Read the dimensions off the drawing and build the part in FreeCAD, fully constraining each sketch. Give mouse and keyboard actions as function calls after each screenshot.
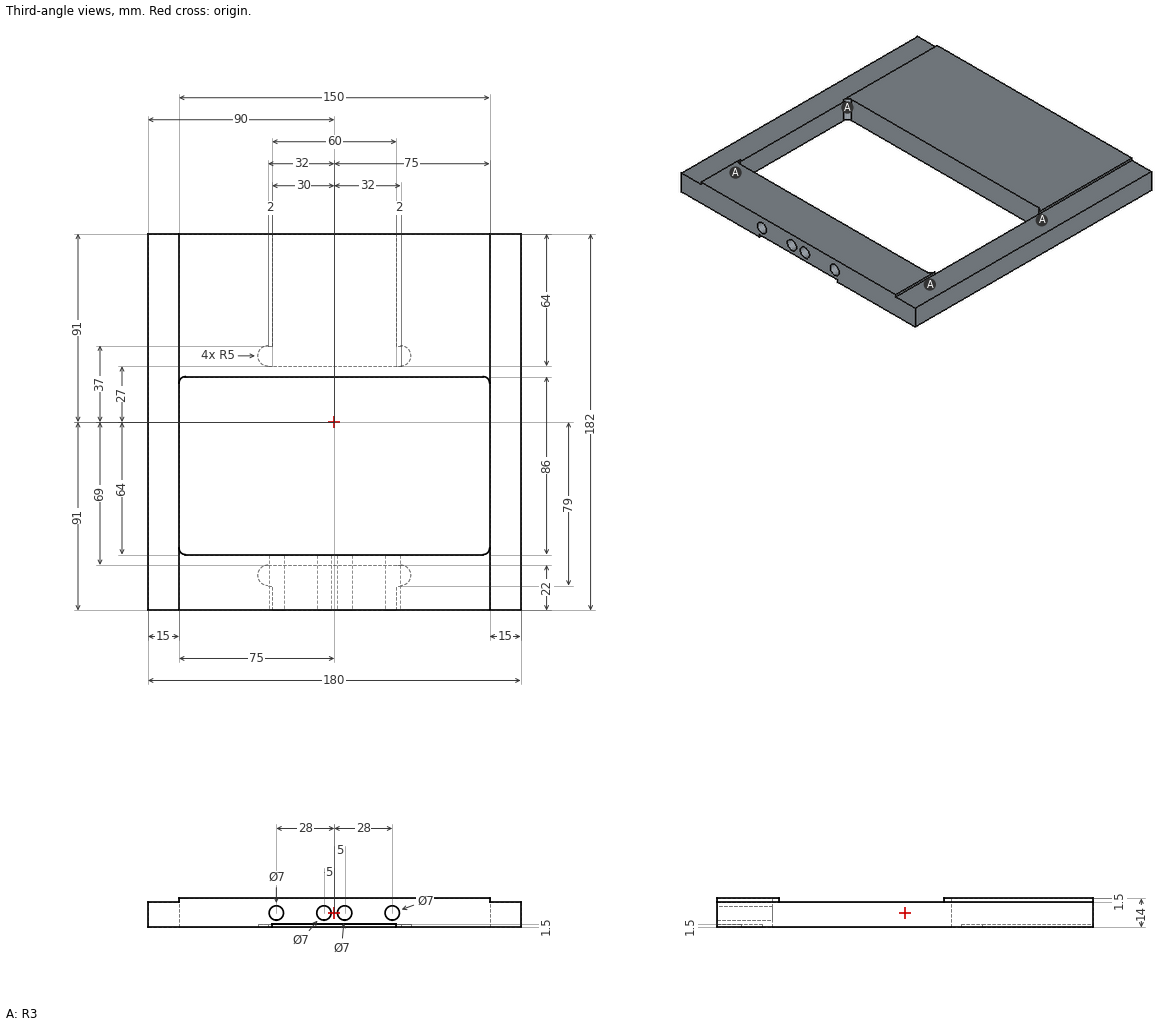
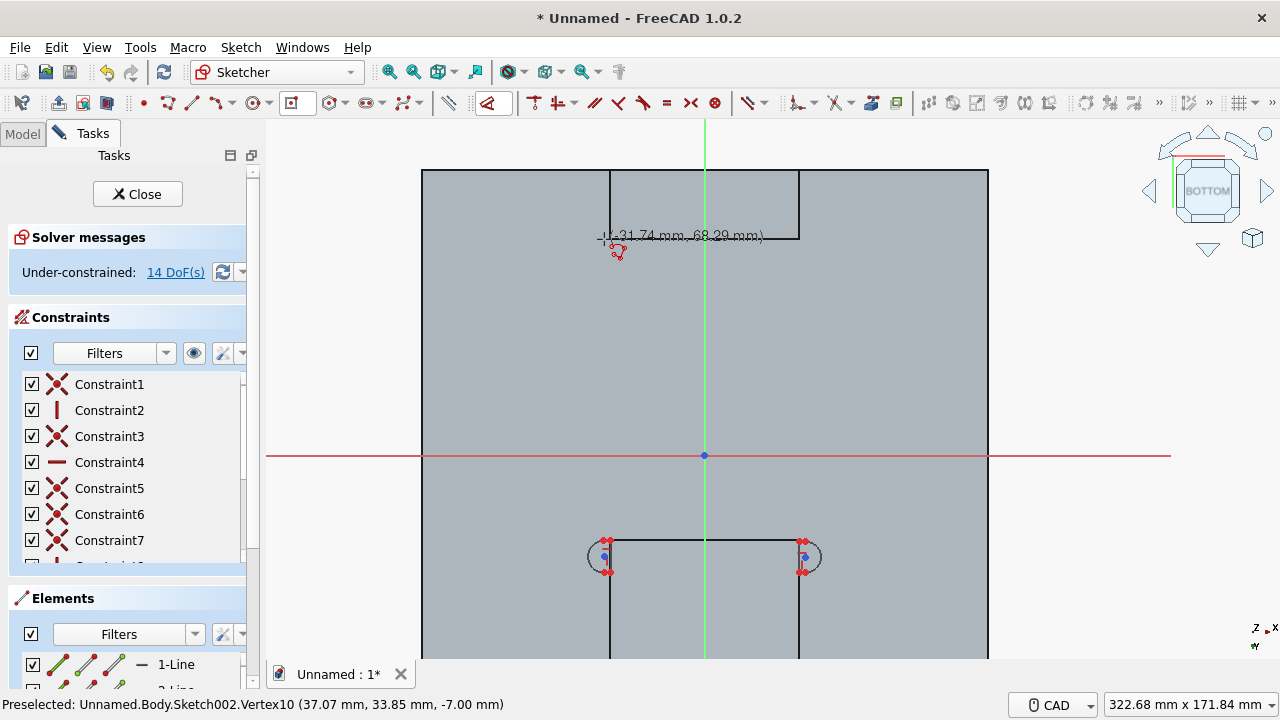
scroll(610, 239, up, 5)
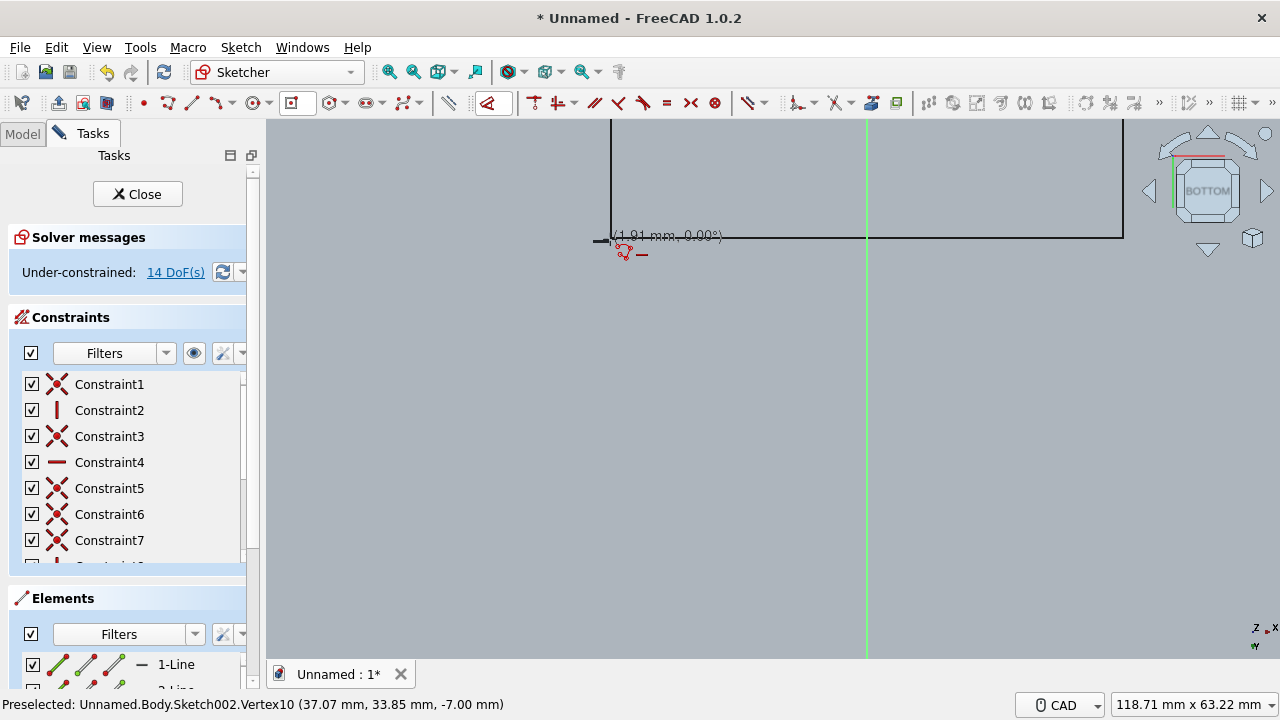
click(611, 239)
click(611, 153)
click(594, 153)
right_click(594, 153)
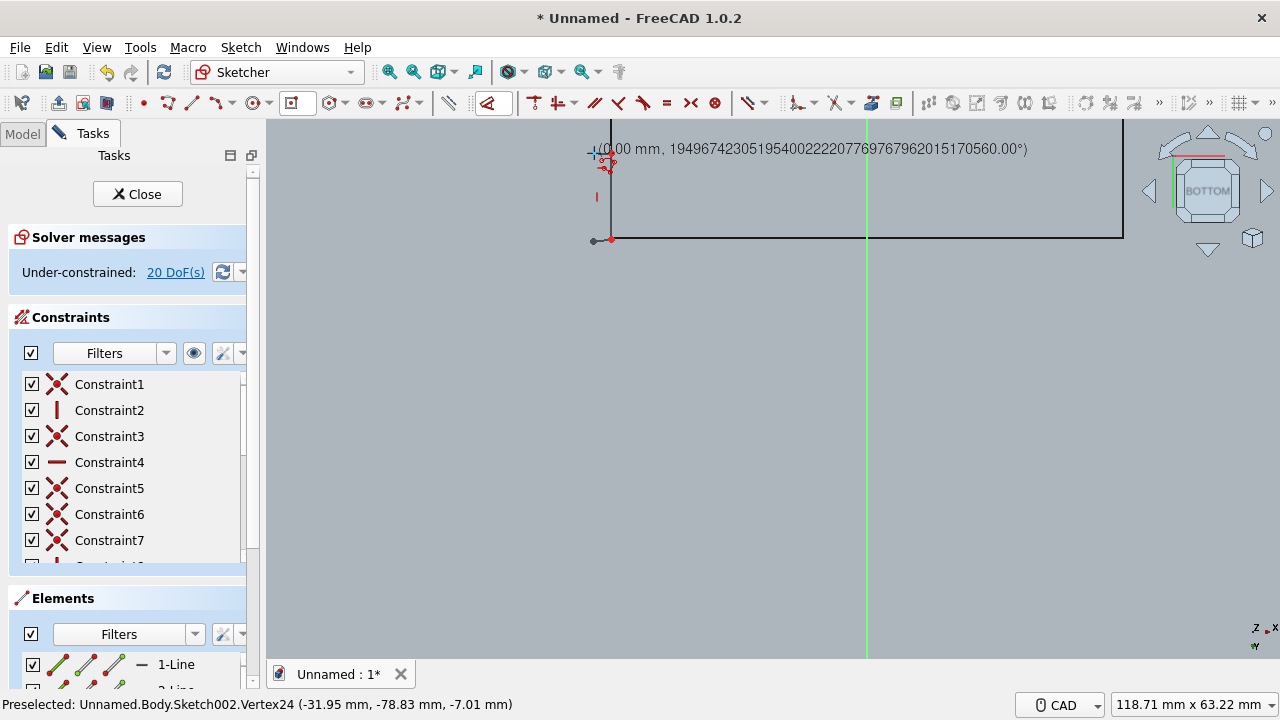
key(g)
key(3)
key(a)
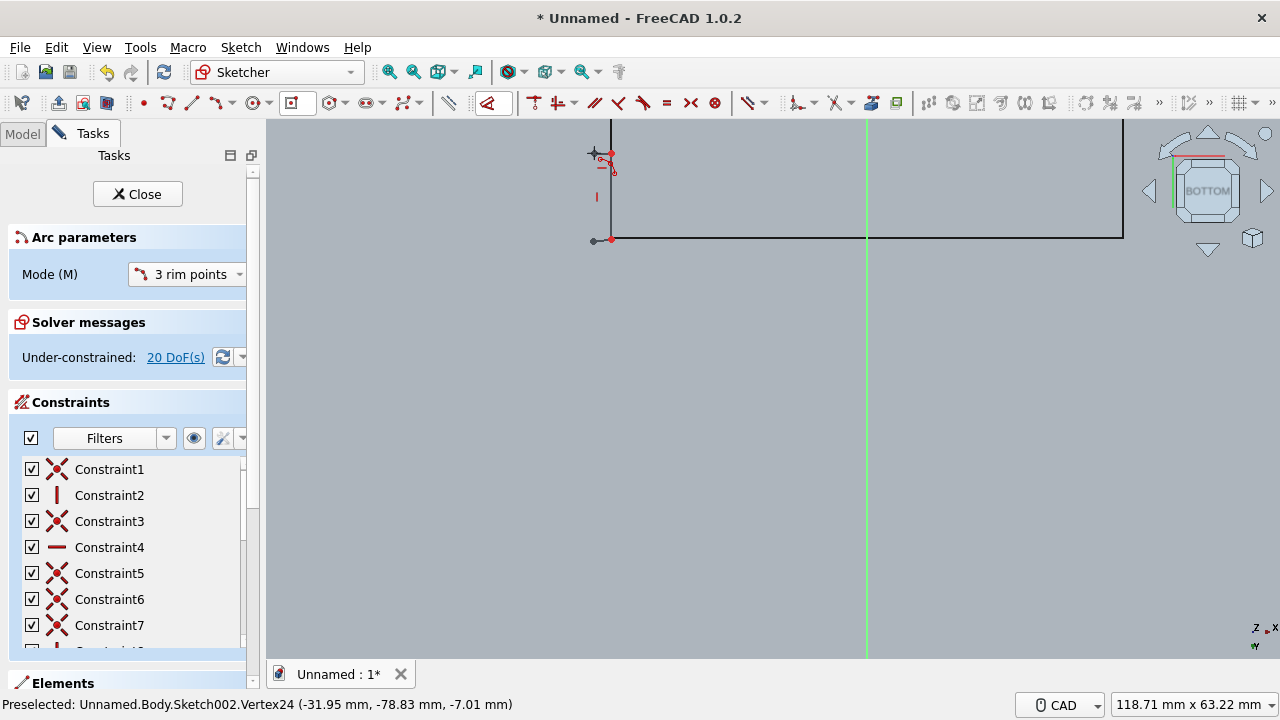
scroll(594, 153, up, 4)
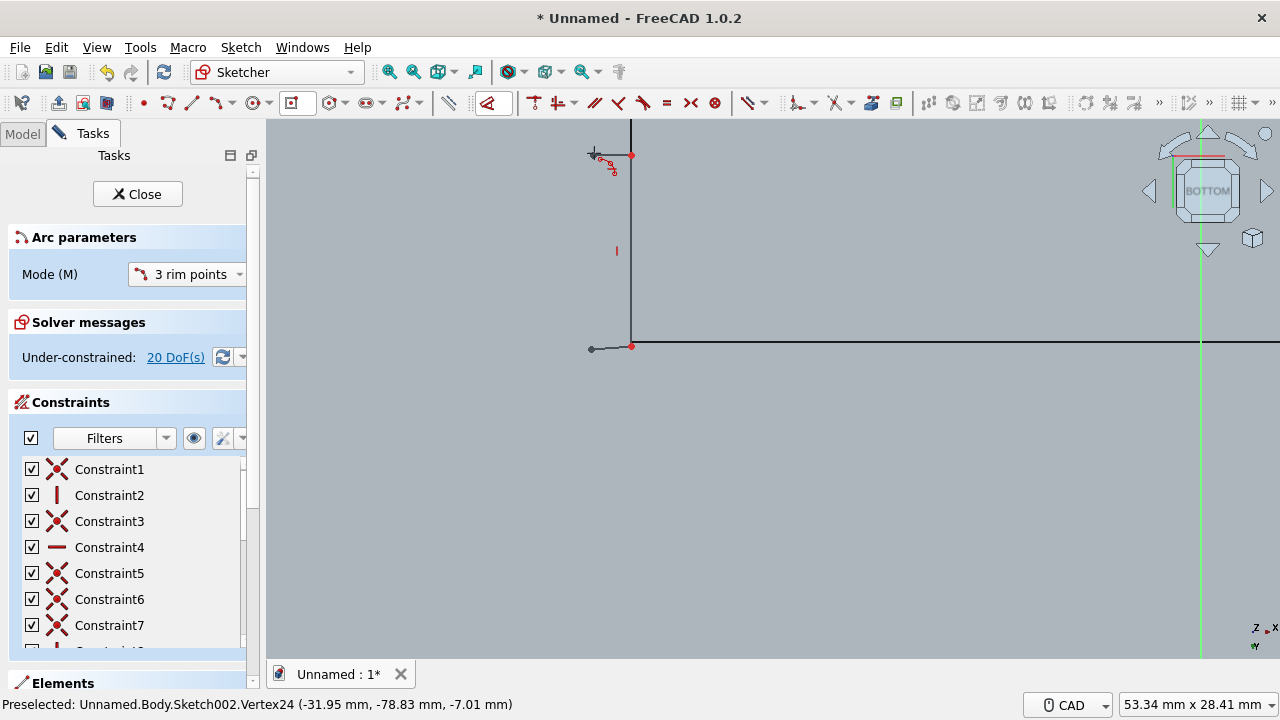
click(594, 155)
click(592, 350)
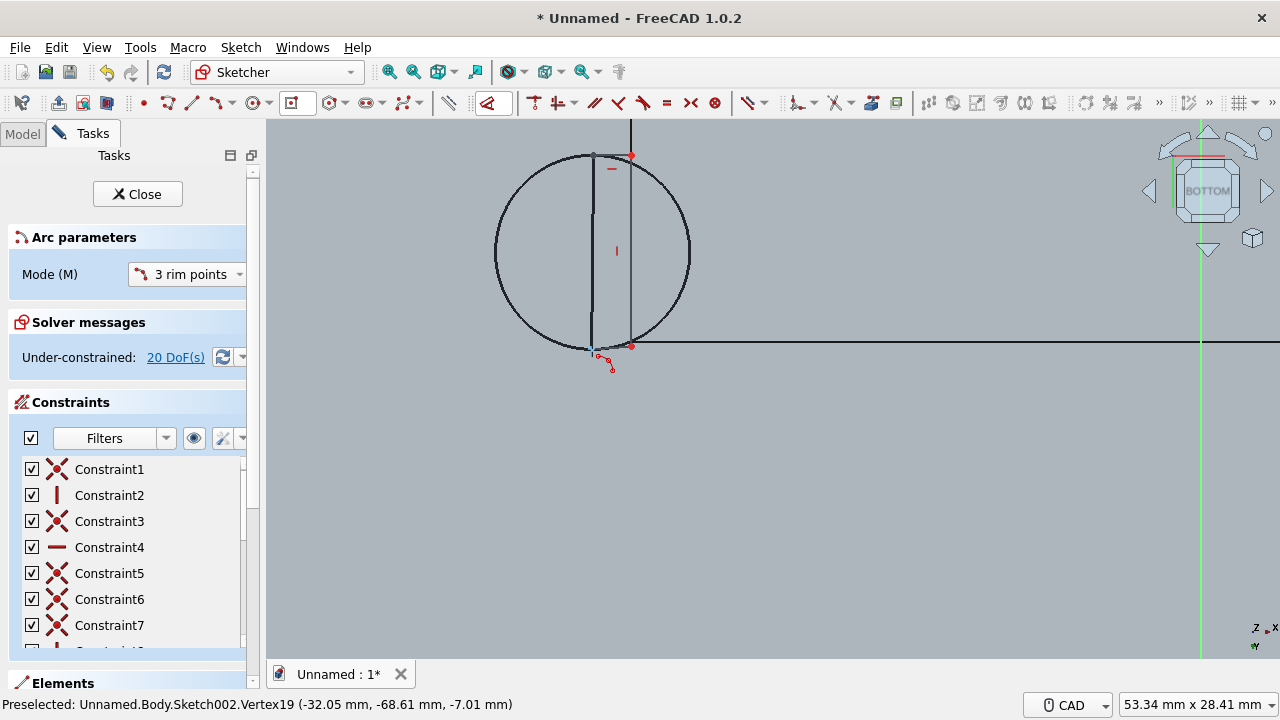
scroll(606, 218, down, 9)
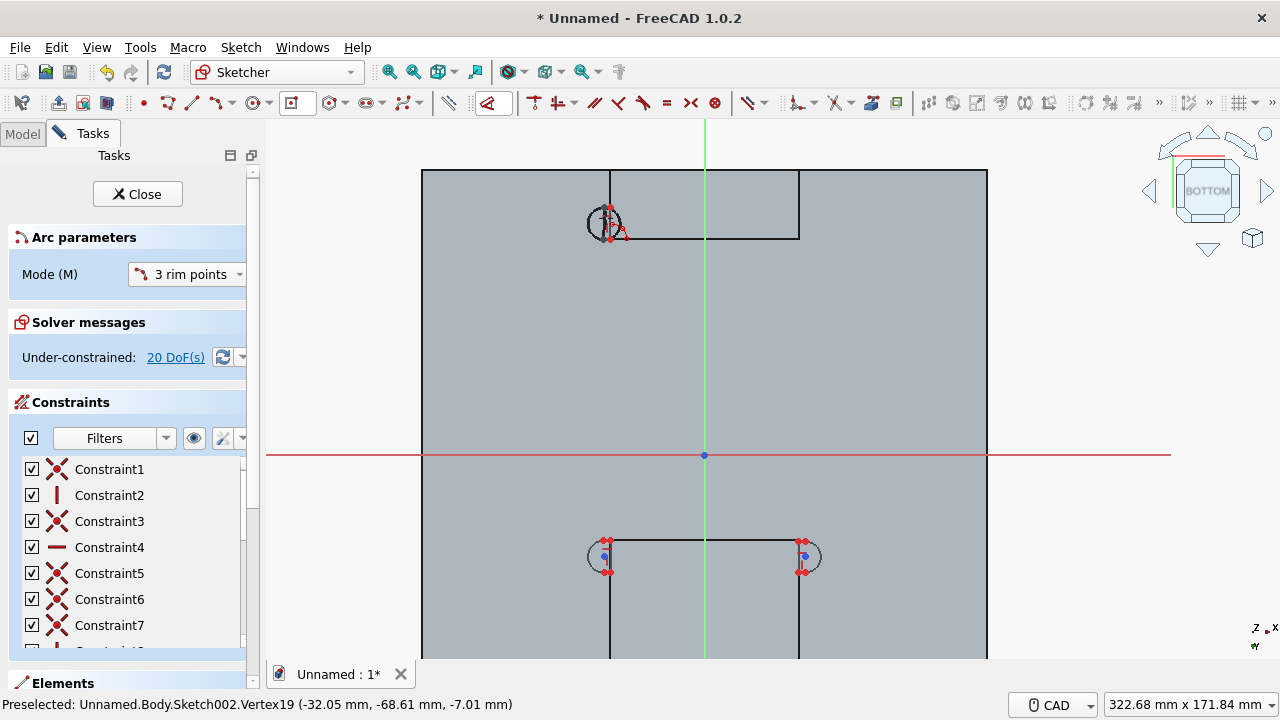
click(588, 223)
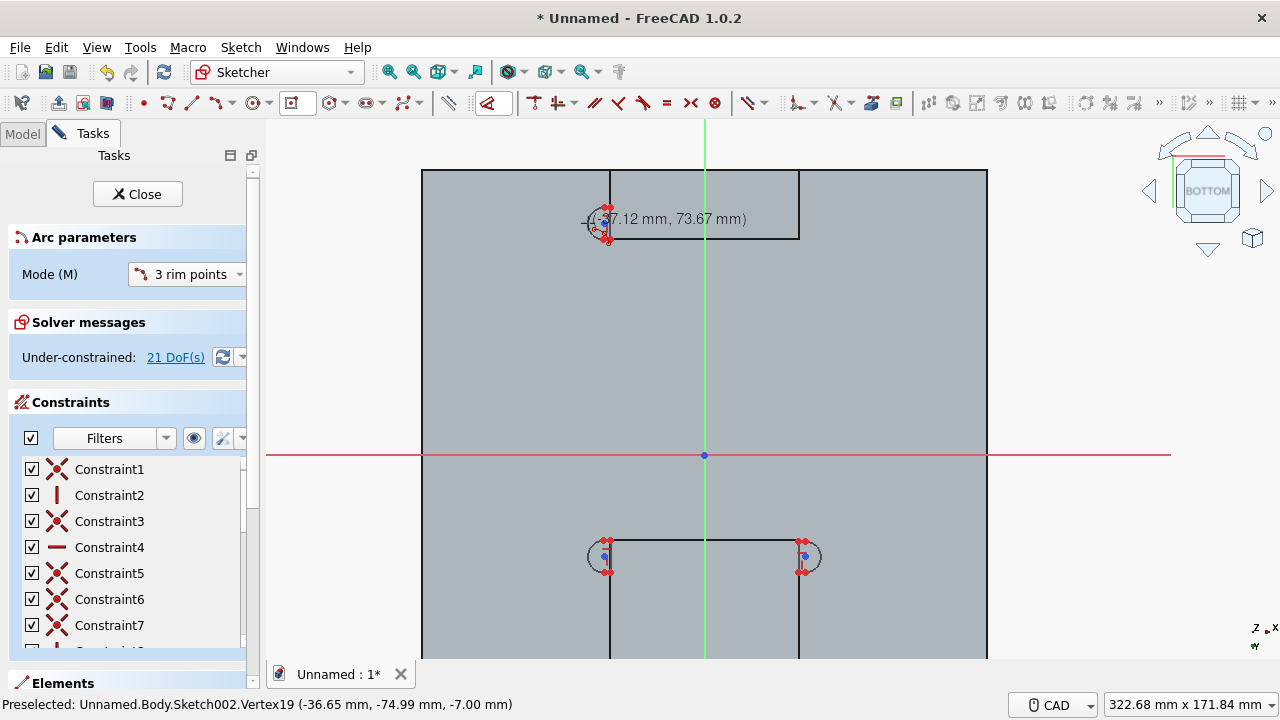
key(g)
key(m)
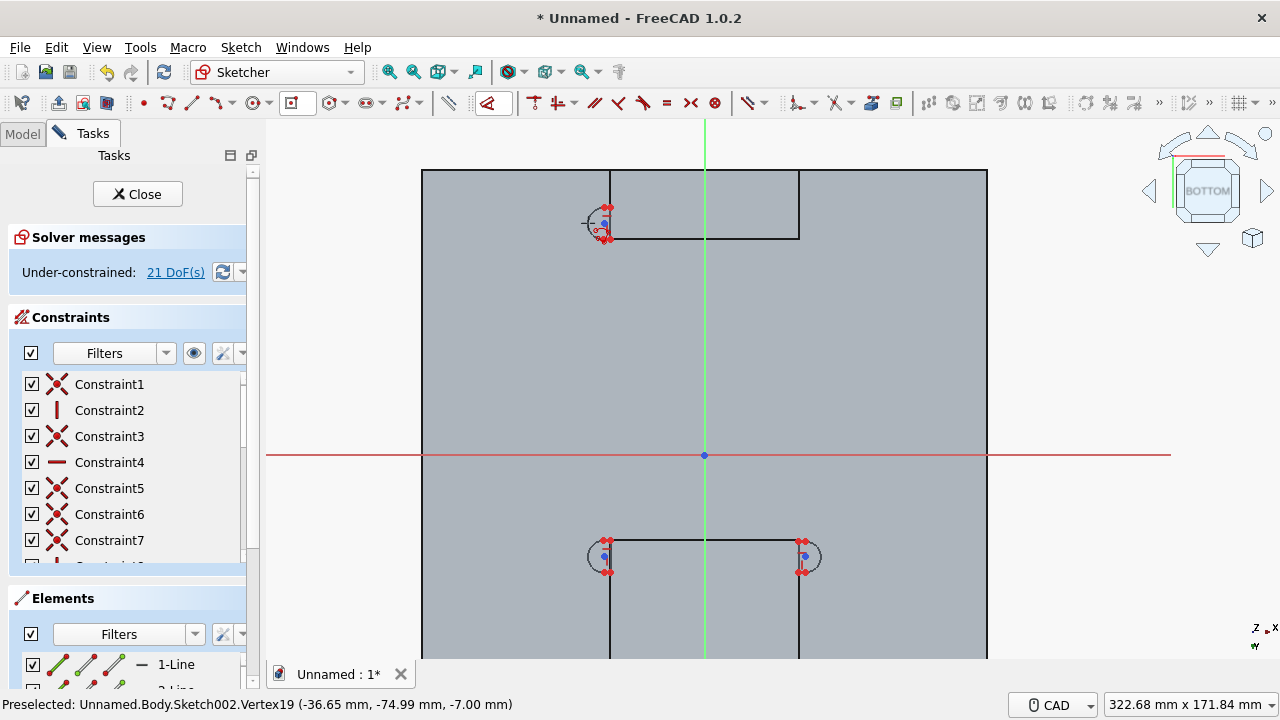
click(805, 207)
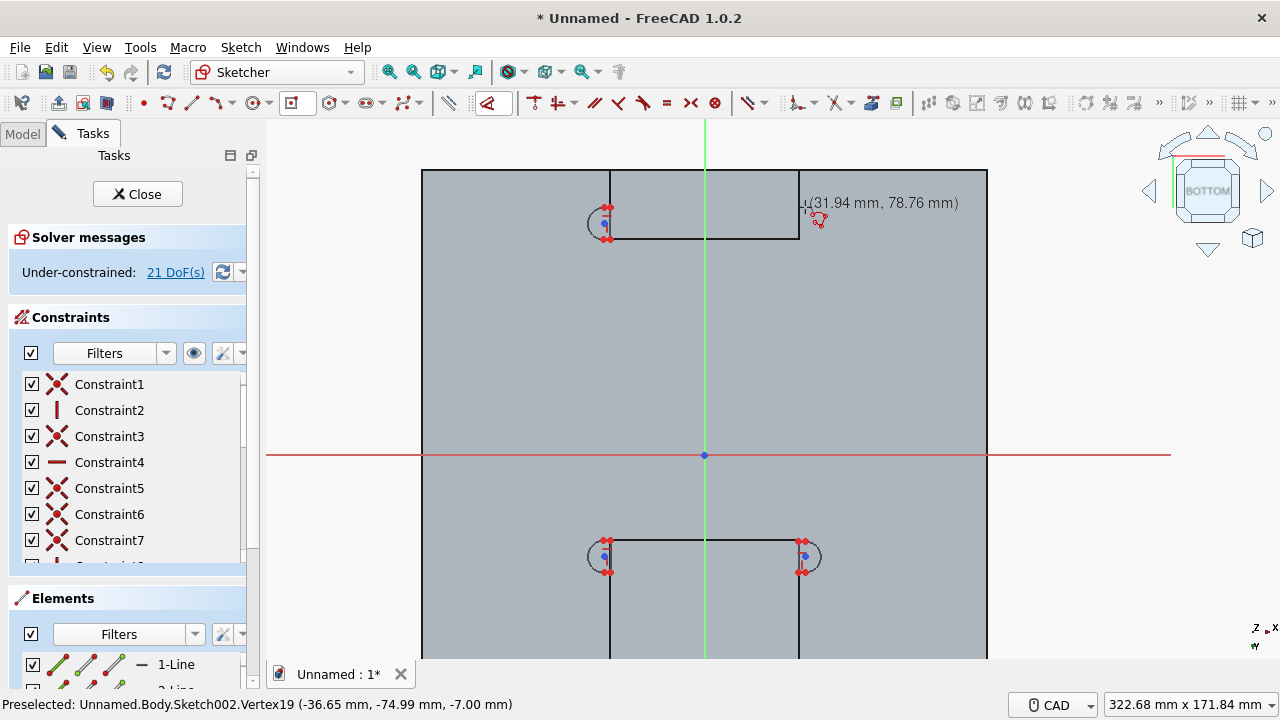
scroll(799, 207, up, 5)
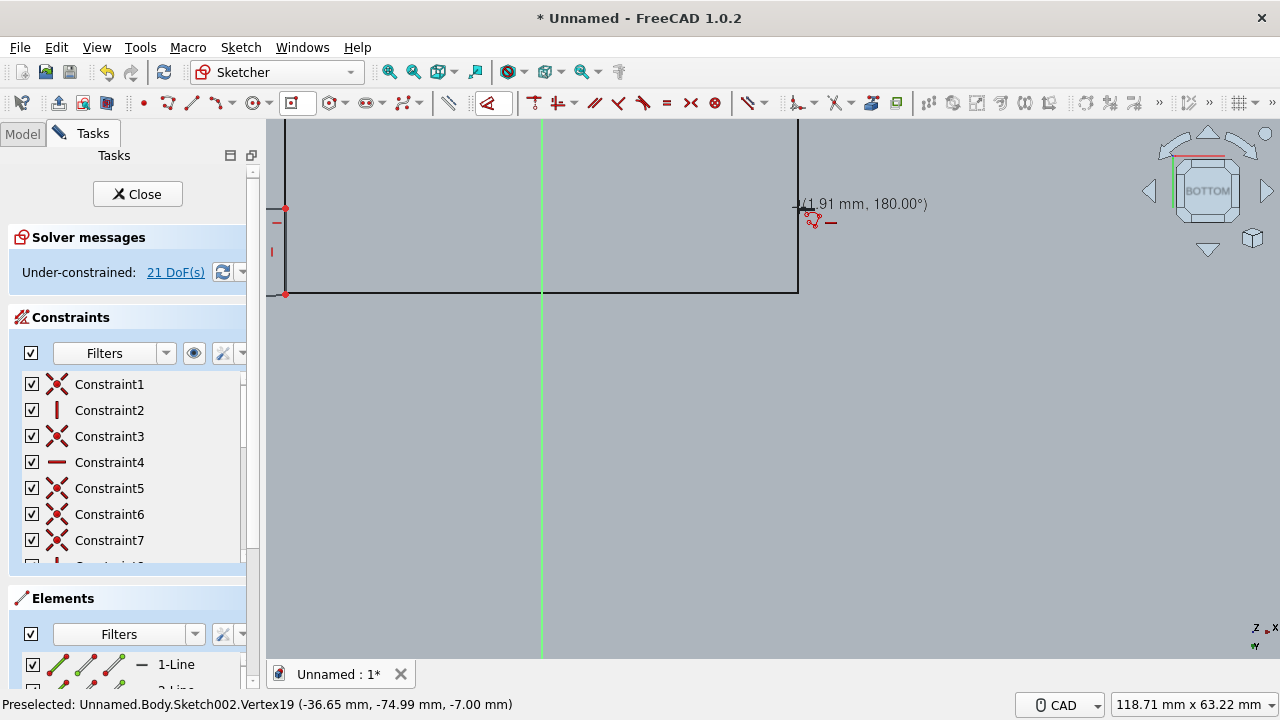
click(798, 207)
click(798, 293)
click(815, 293)
right_click(815, 293)